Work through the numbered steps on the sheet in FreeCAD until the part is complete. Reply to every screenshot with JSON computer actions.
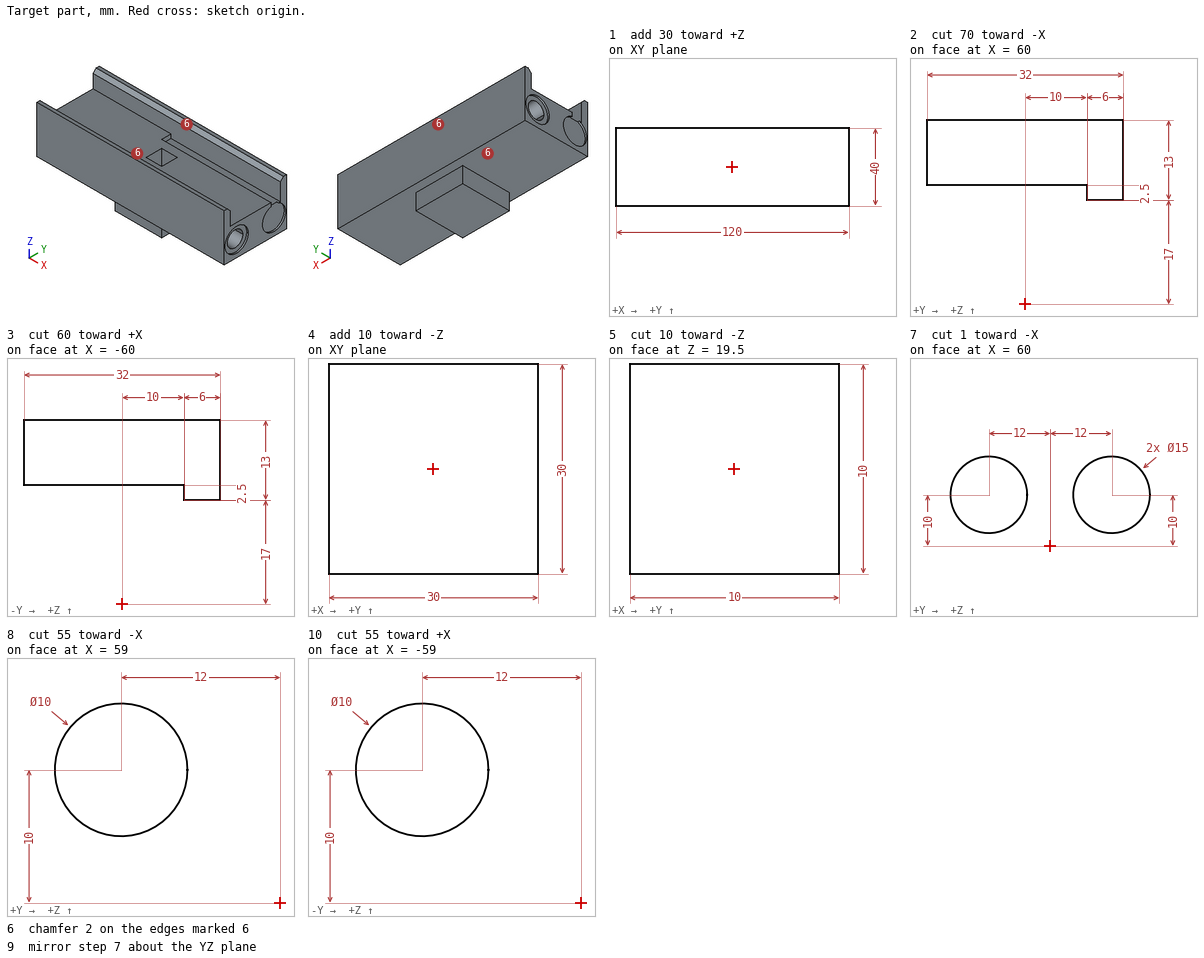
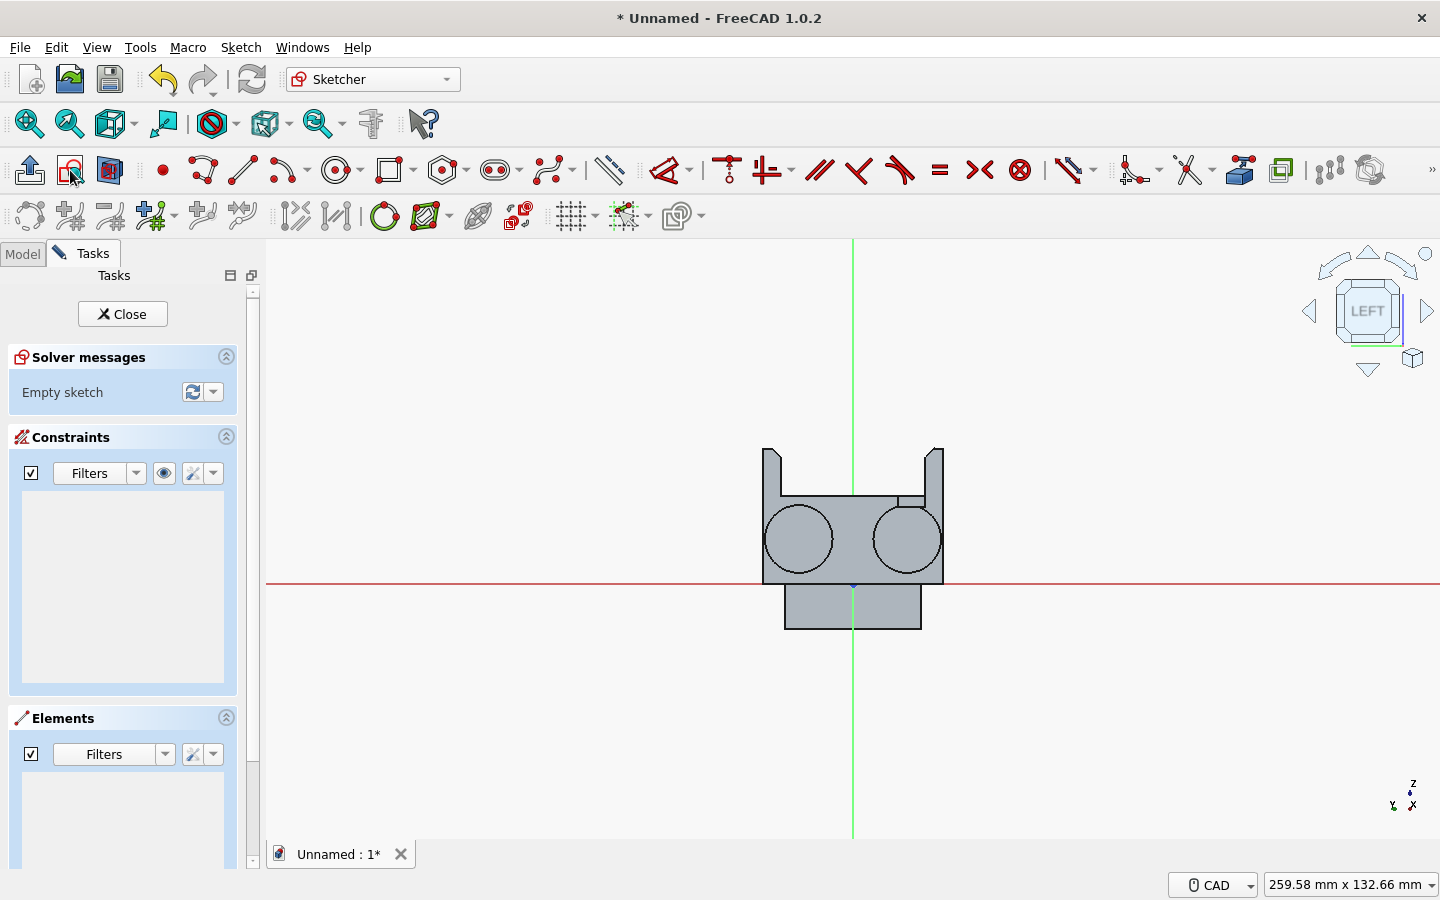
{"action": "key", "text": "q s"}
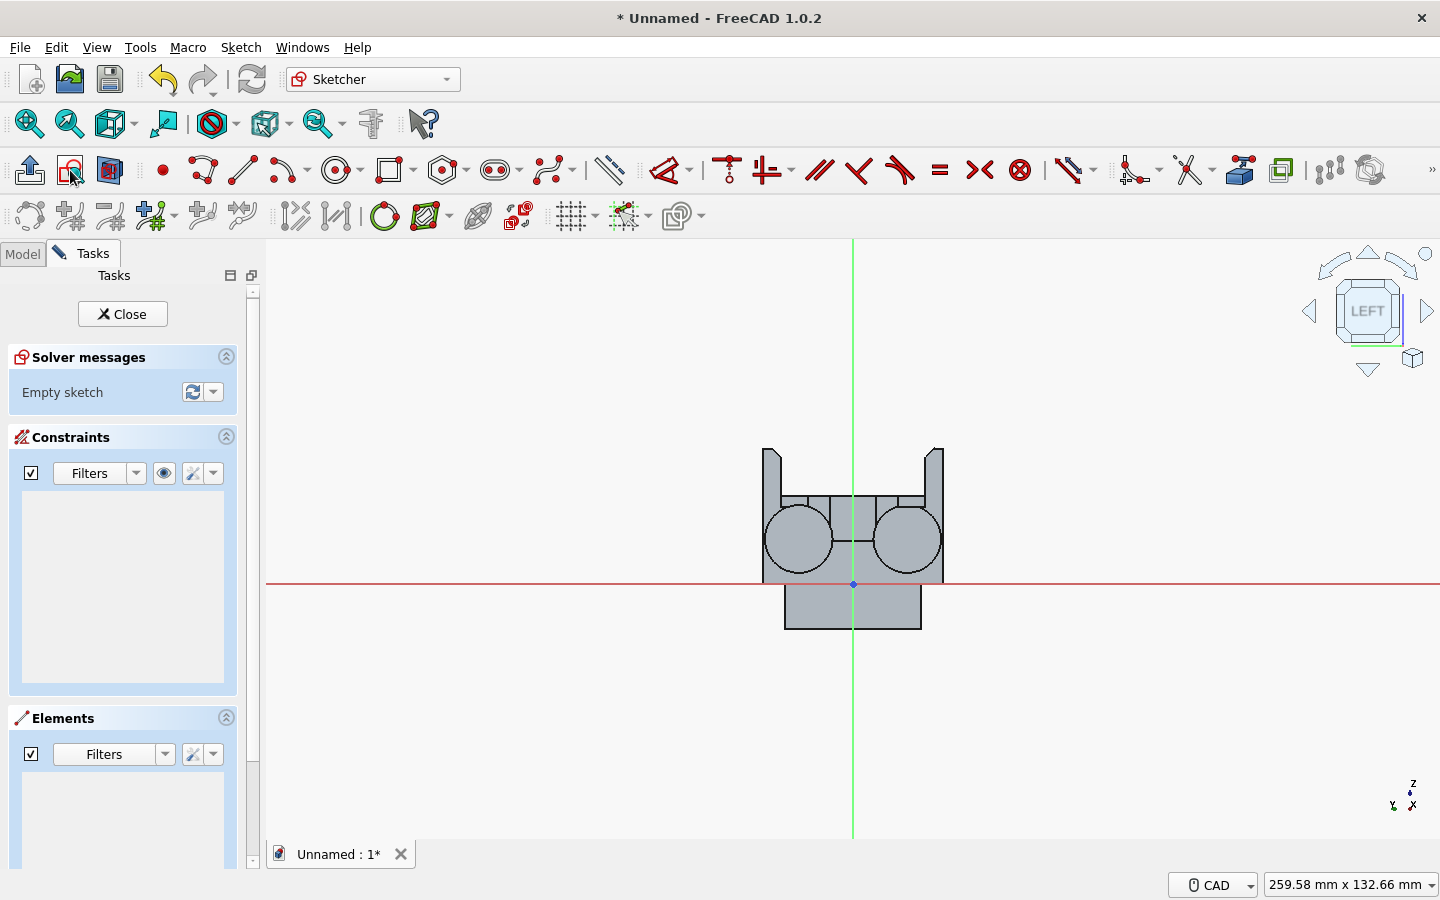
{"action": "scroll", "coordinate": [821, 553], "scroll_direction": "up", "scroll_amount": 9}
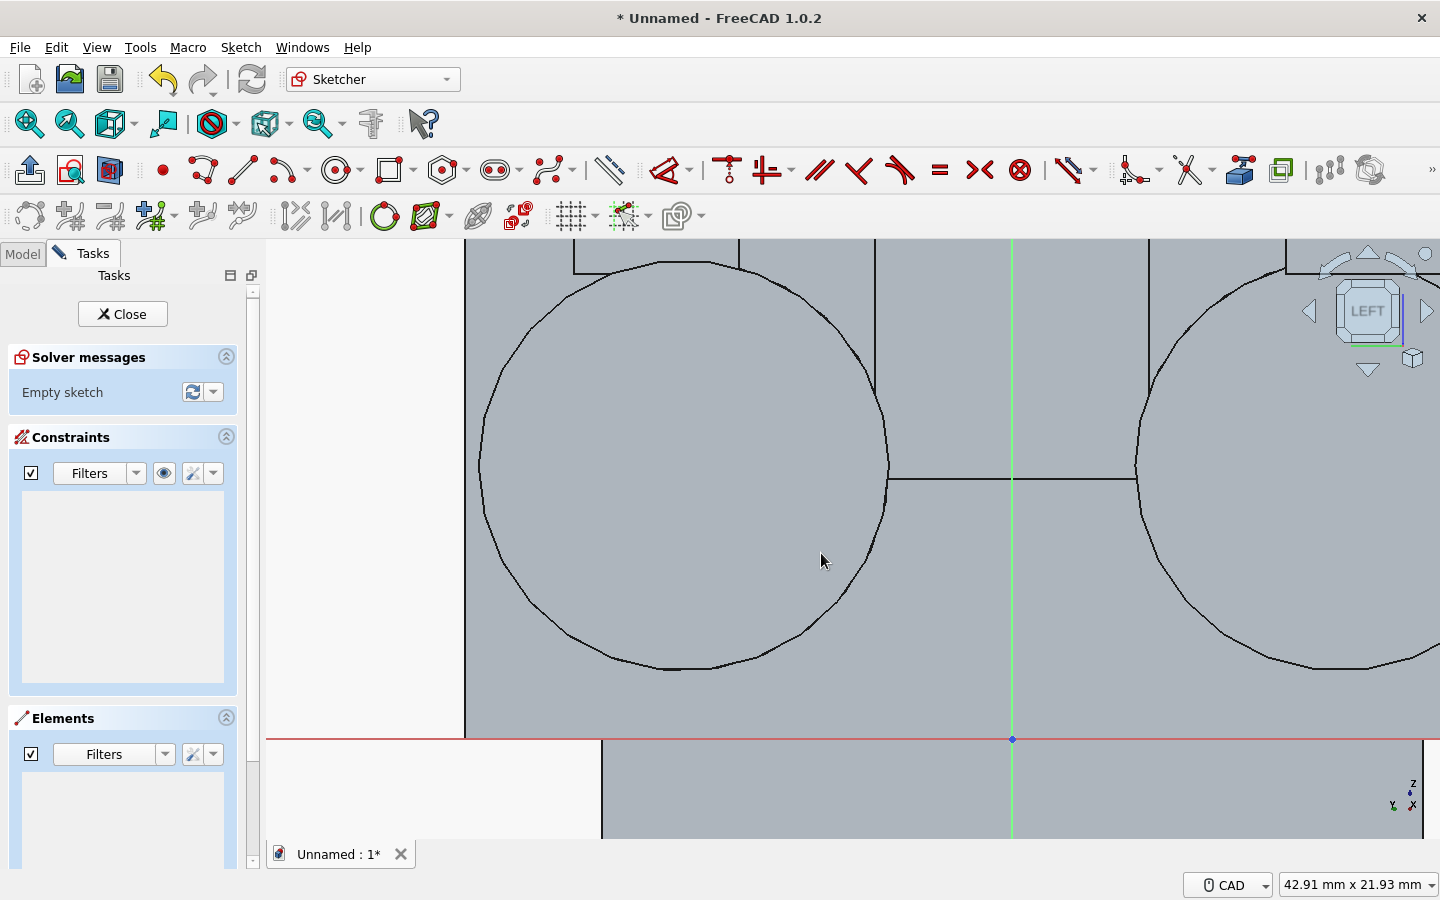
{"action": "key", "text": "g c"}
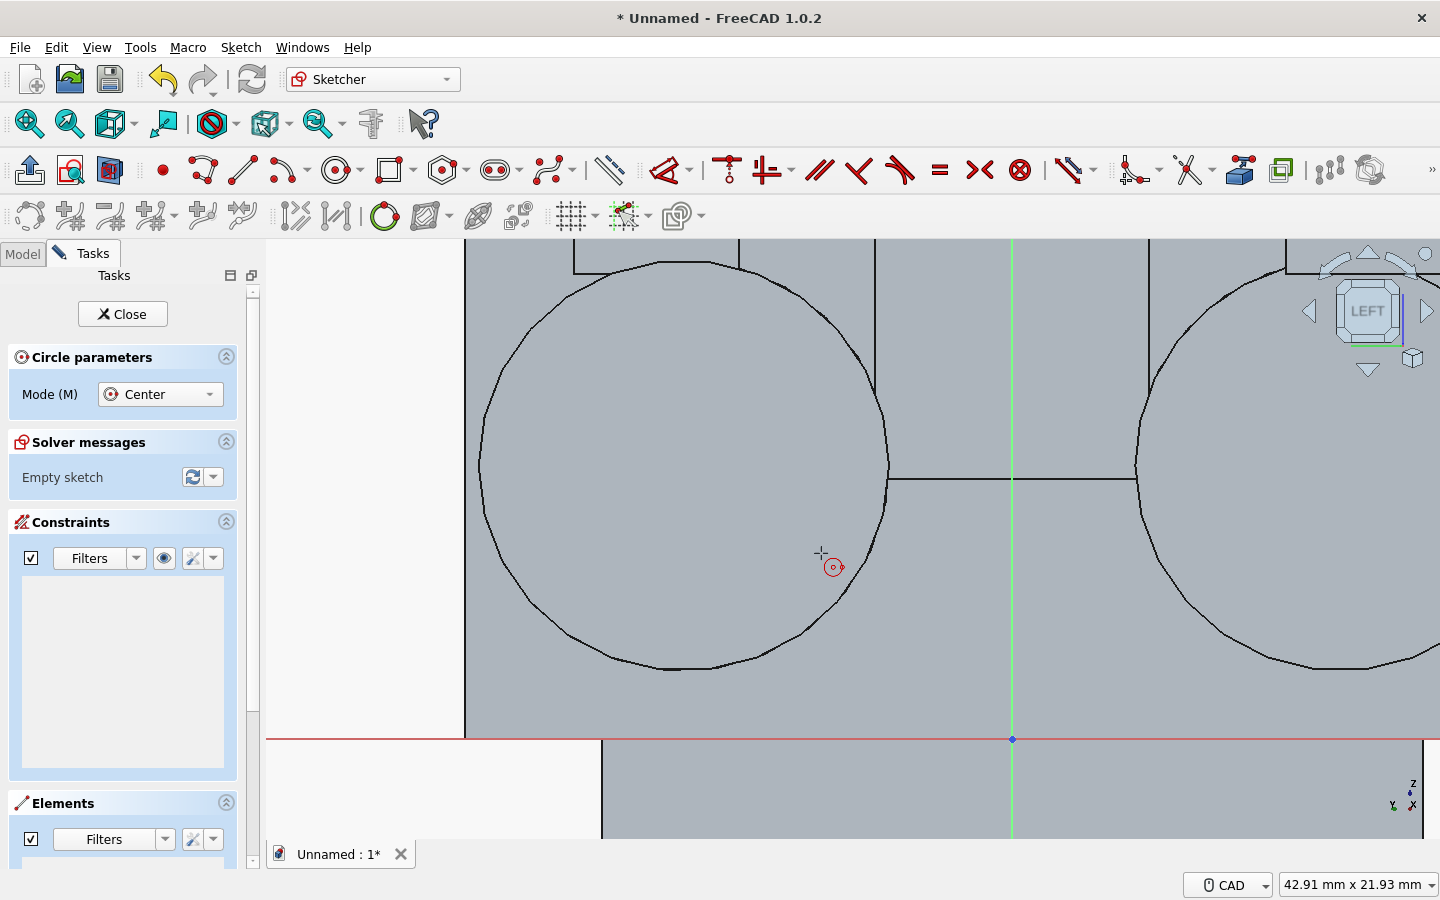
{"action": "left_click", "coordinate": [684, 466]}
{"action": "mouse_move", "coordinate": [781, 369]}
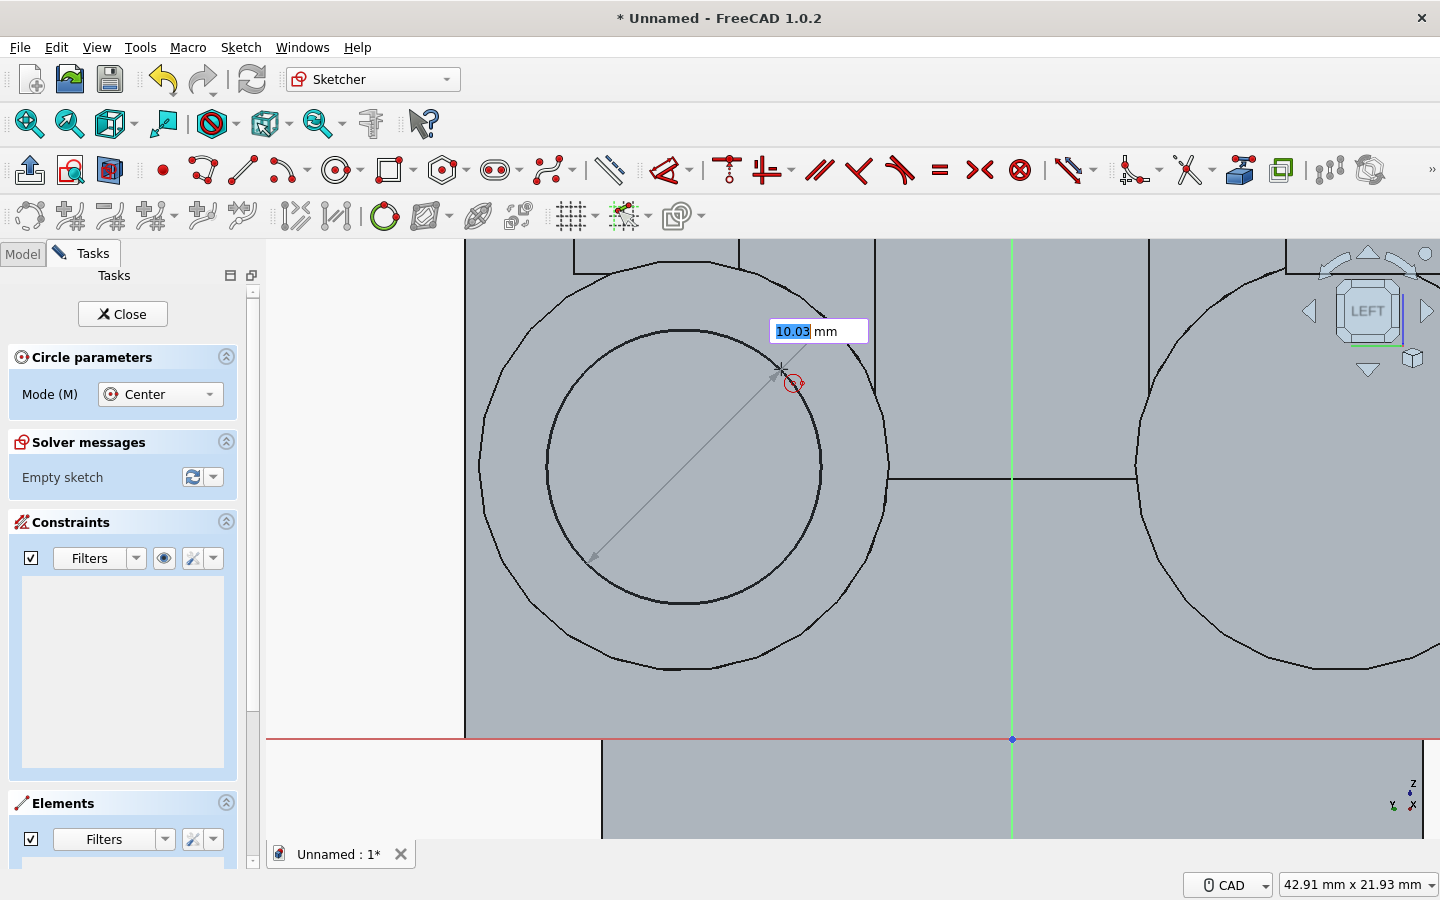
{"action": "type", "text": "10"}
{"action": "key", "text": "Return"}
{"action": "key", "text": "Escape"}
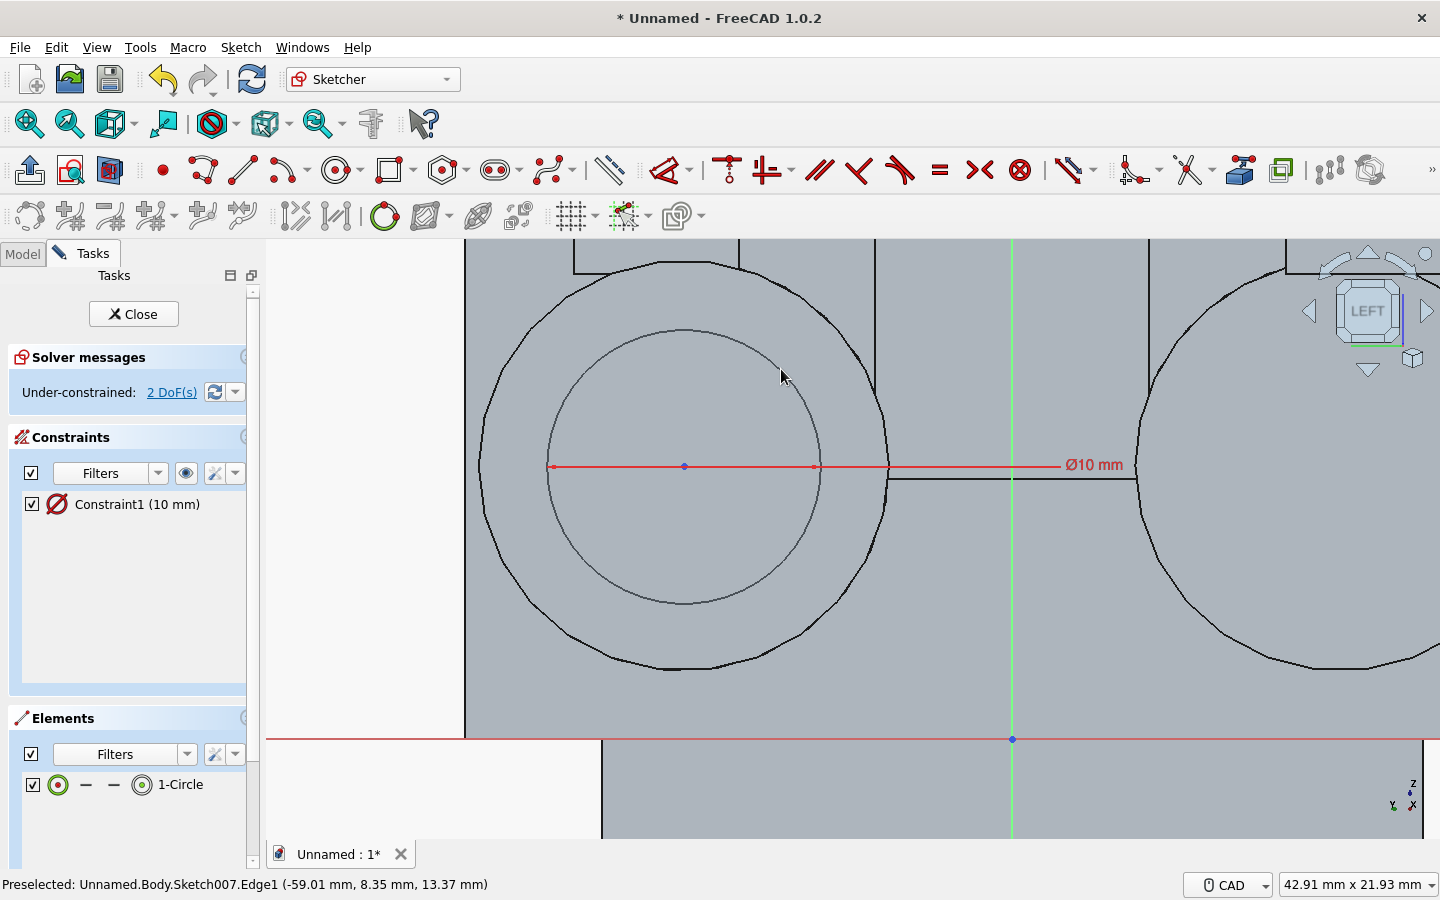
{"action": "left_click", "coordinate": [664, 170]}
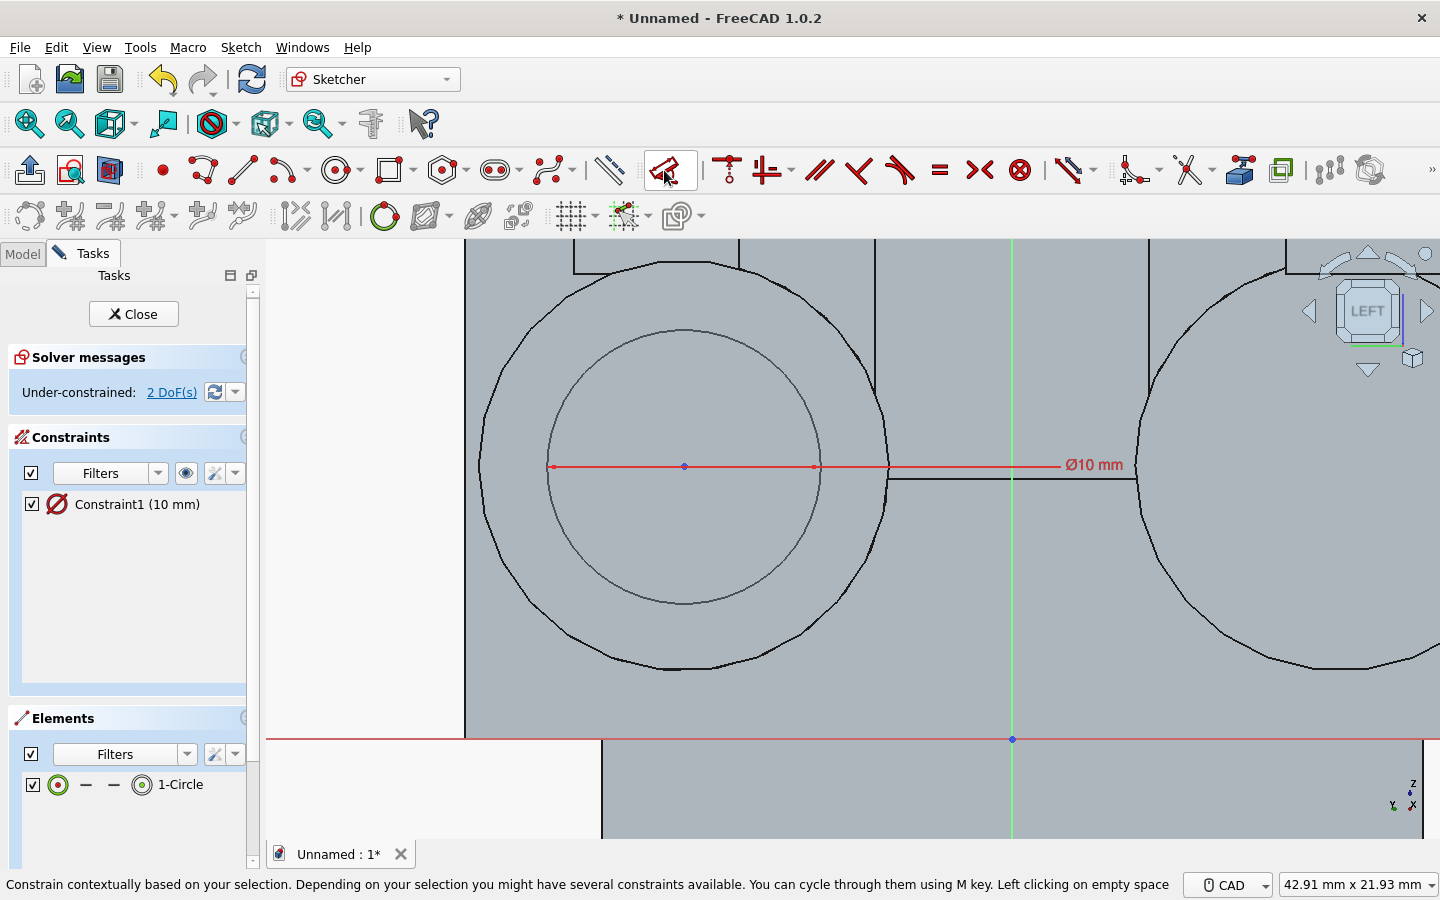
{"action": "left_click", "coordinate": [684, 467]}
{"action": "left_click", "coordinate": [848, 773]}